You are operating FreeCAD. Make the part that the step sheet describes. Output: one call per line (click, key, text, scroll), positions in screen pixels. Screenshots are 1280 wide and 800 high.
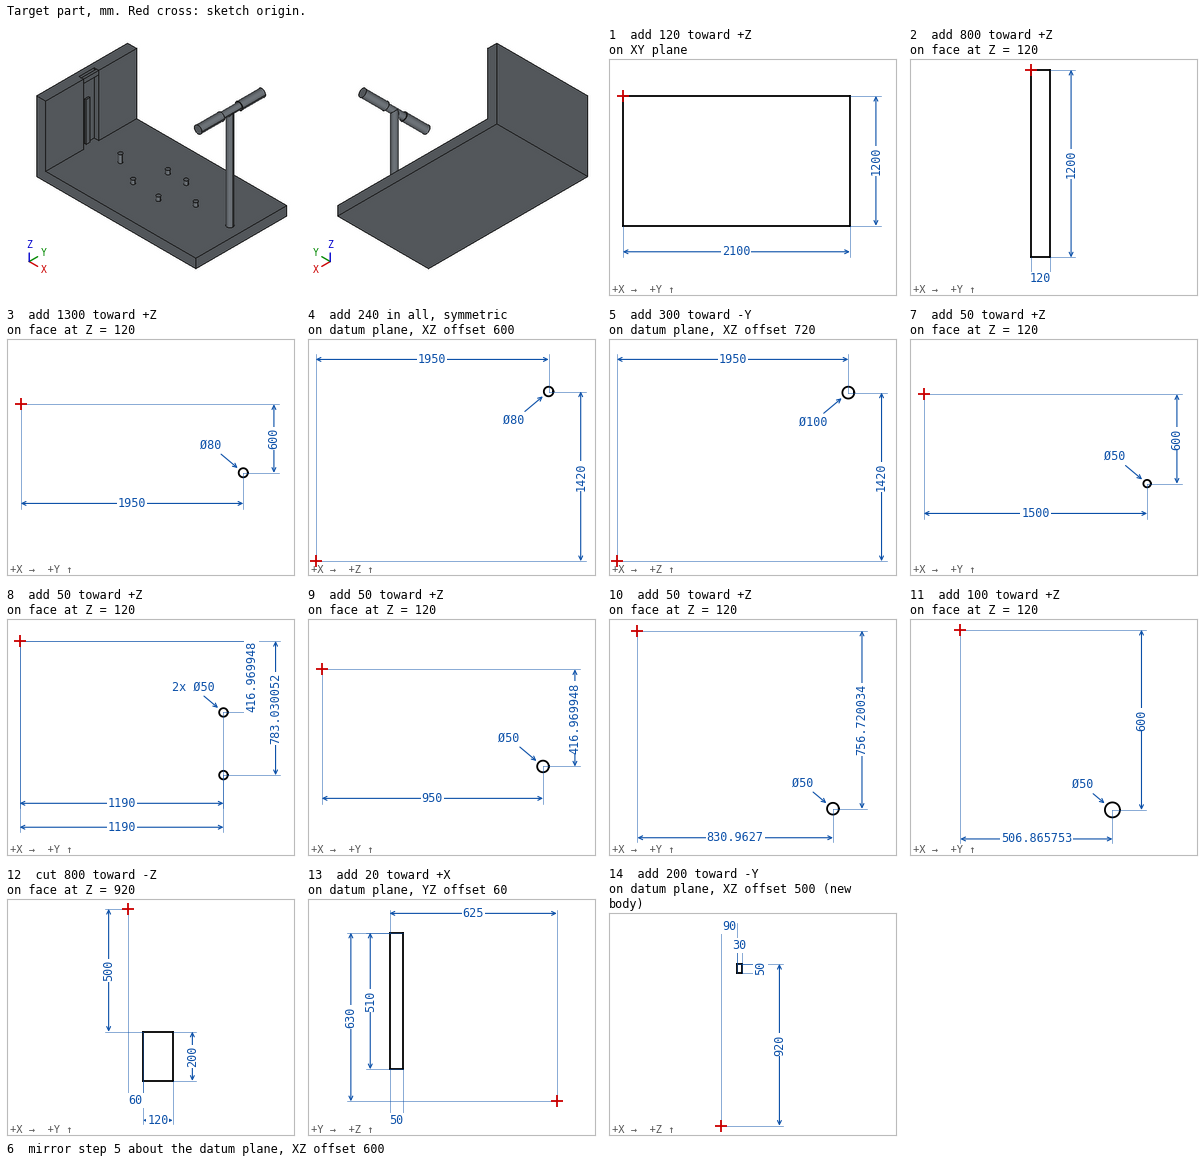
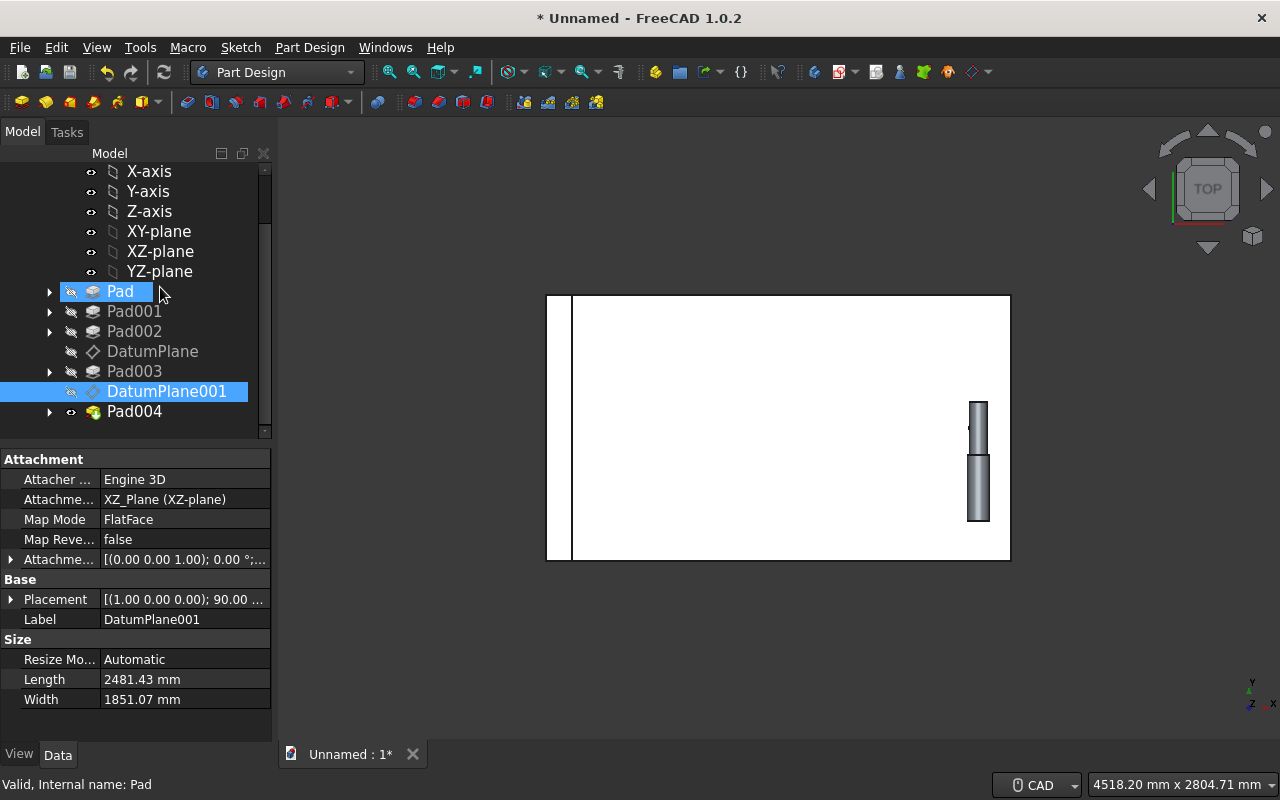
scroll(160, 287, up, 15)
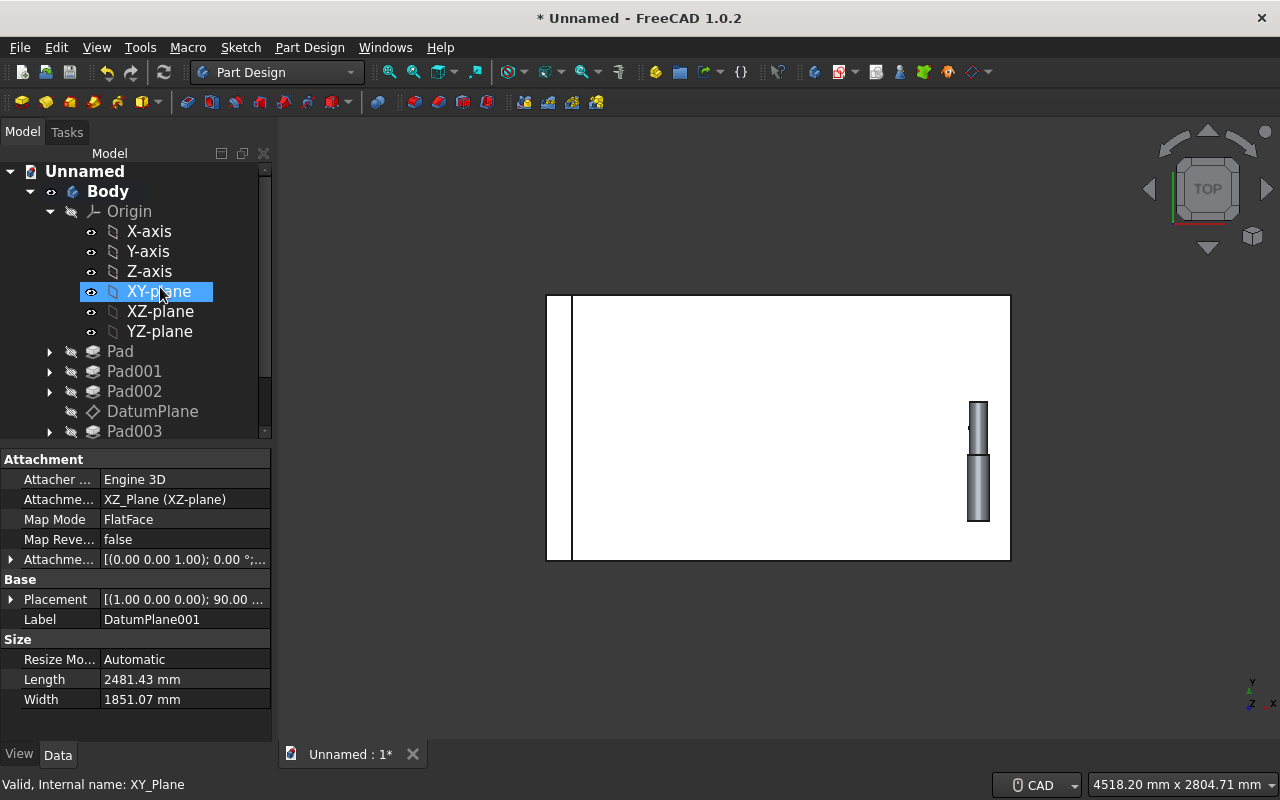
click(136, 312)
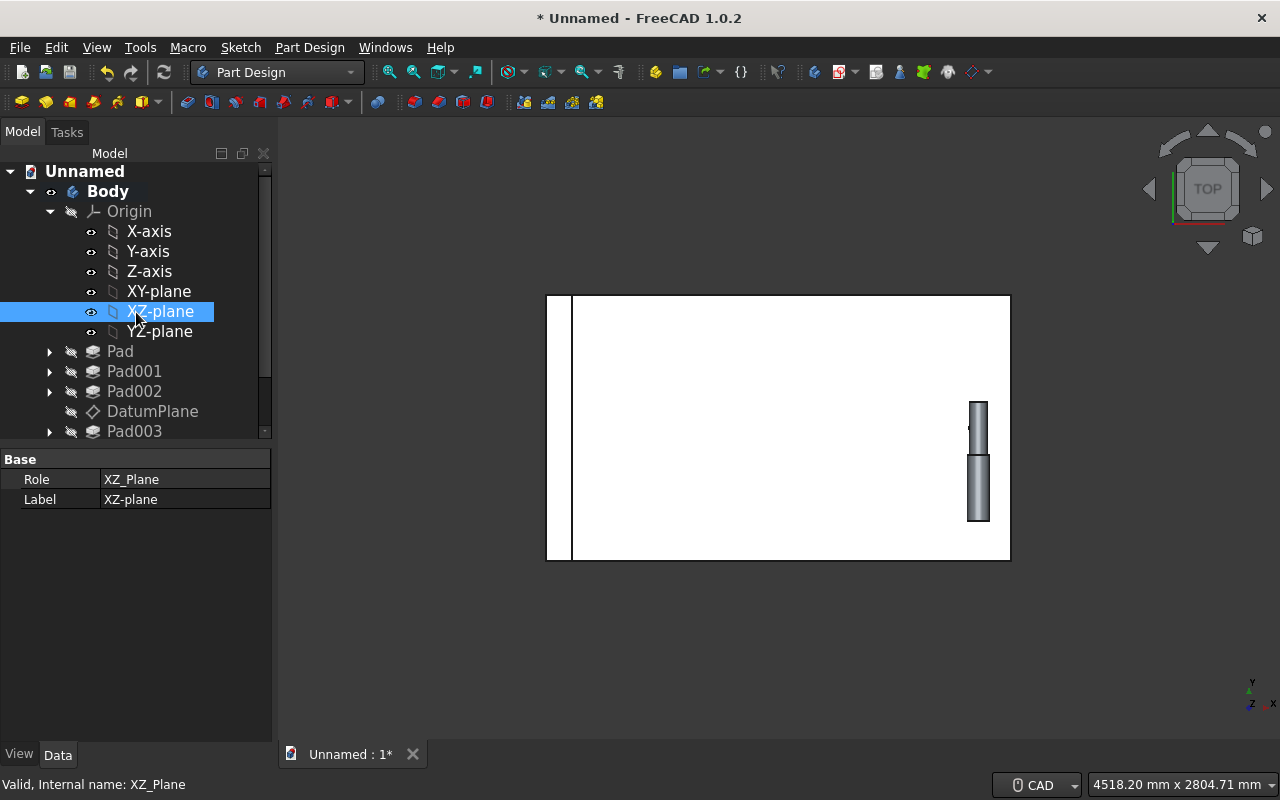
click(972, 72)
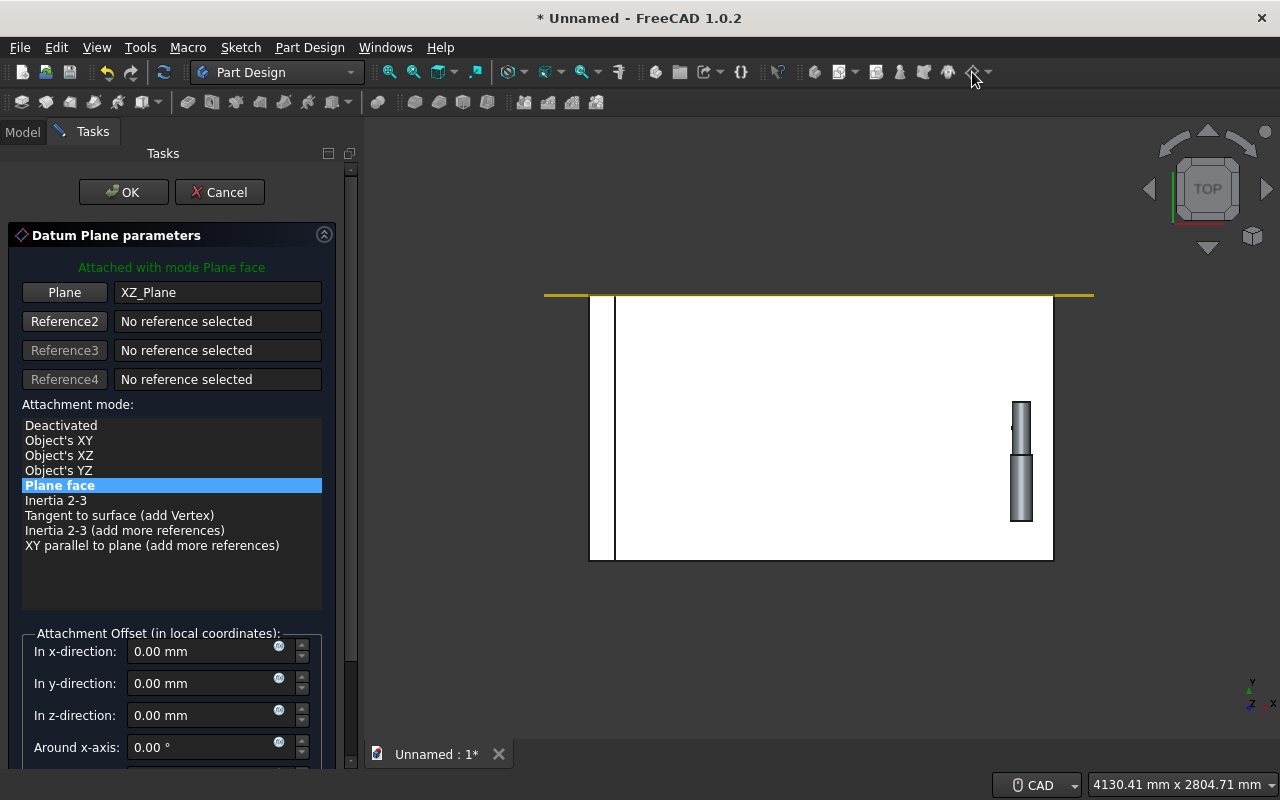
triple_click(210, 715)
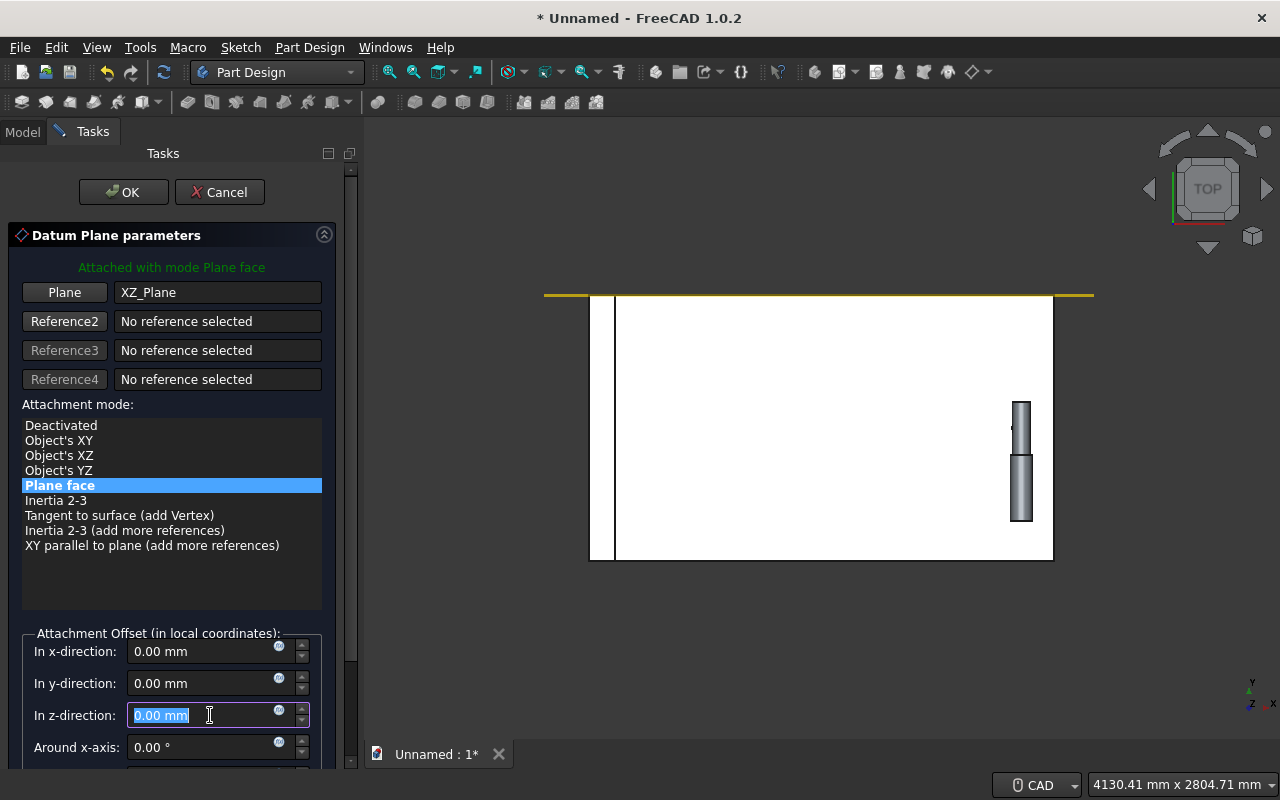
text(600)
key(Tab)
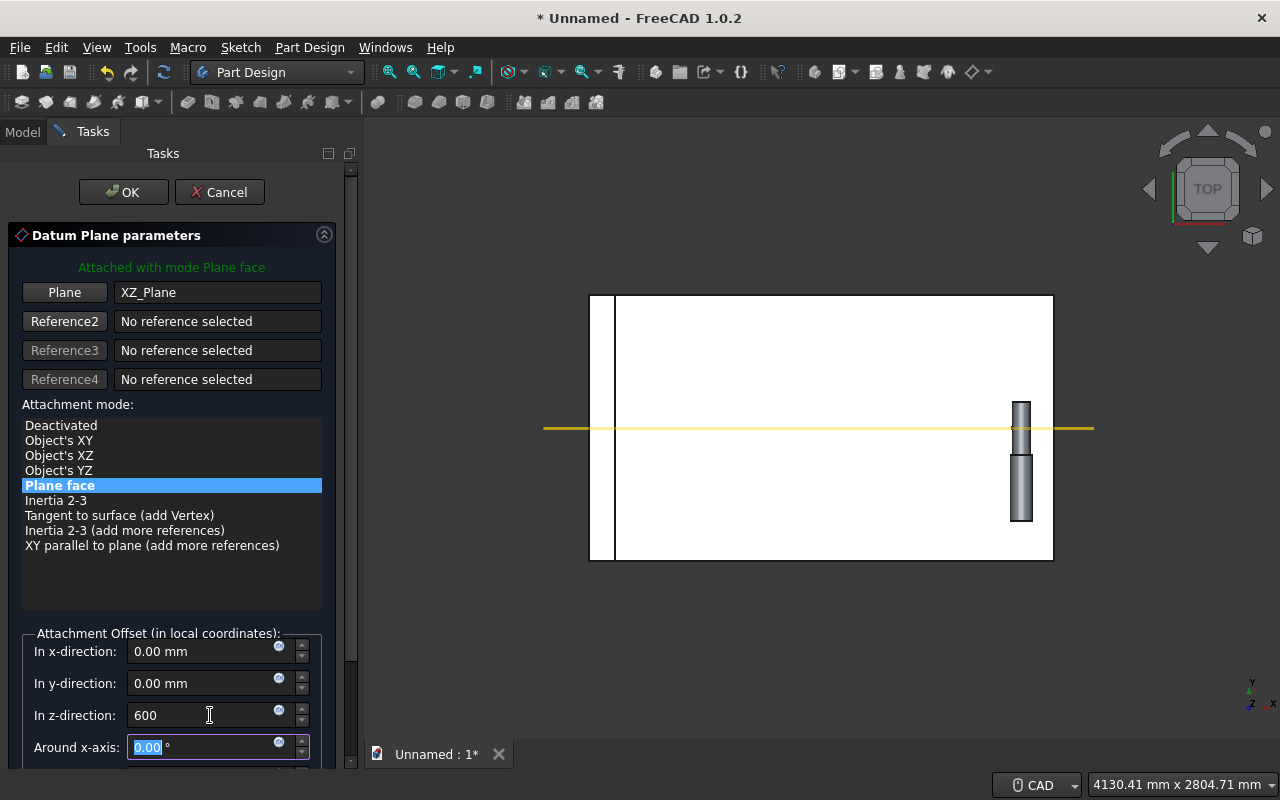
click(124, 192)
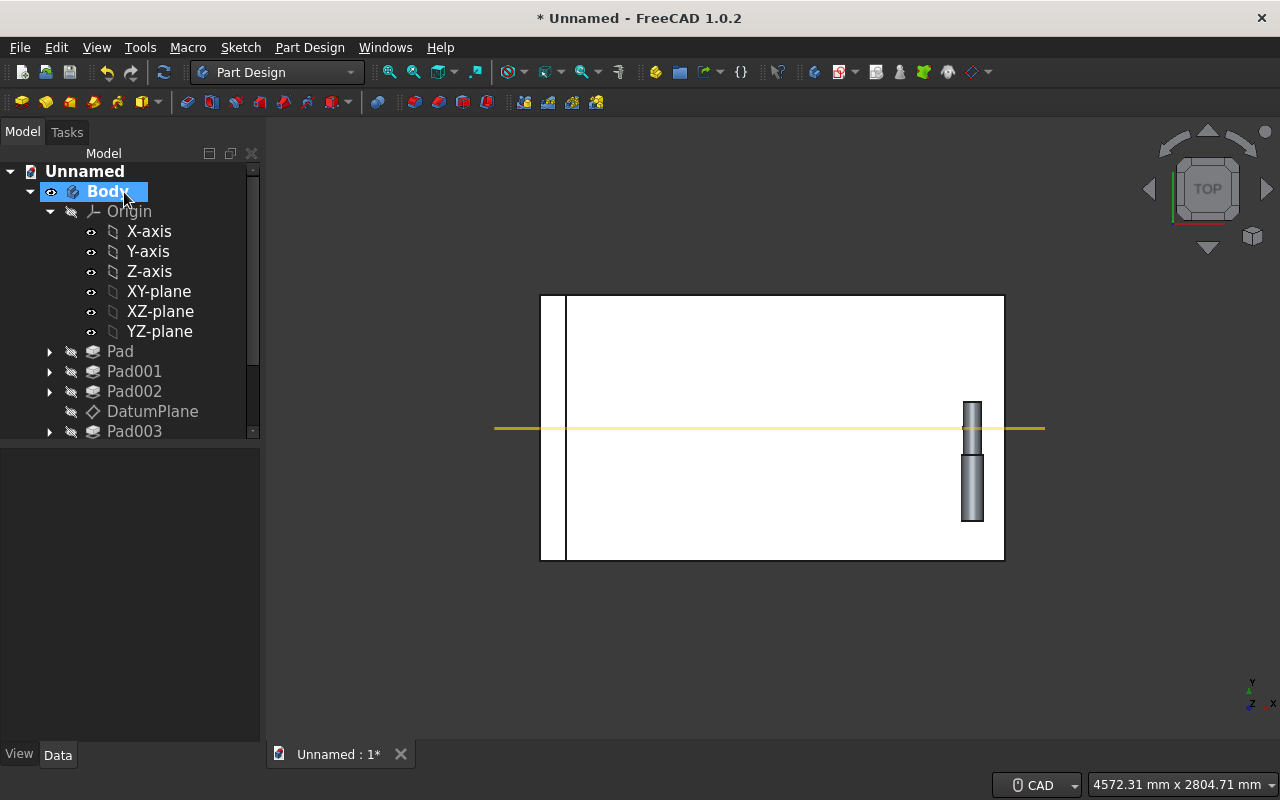
scroll(100, 307, down, 3)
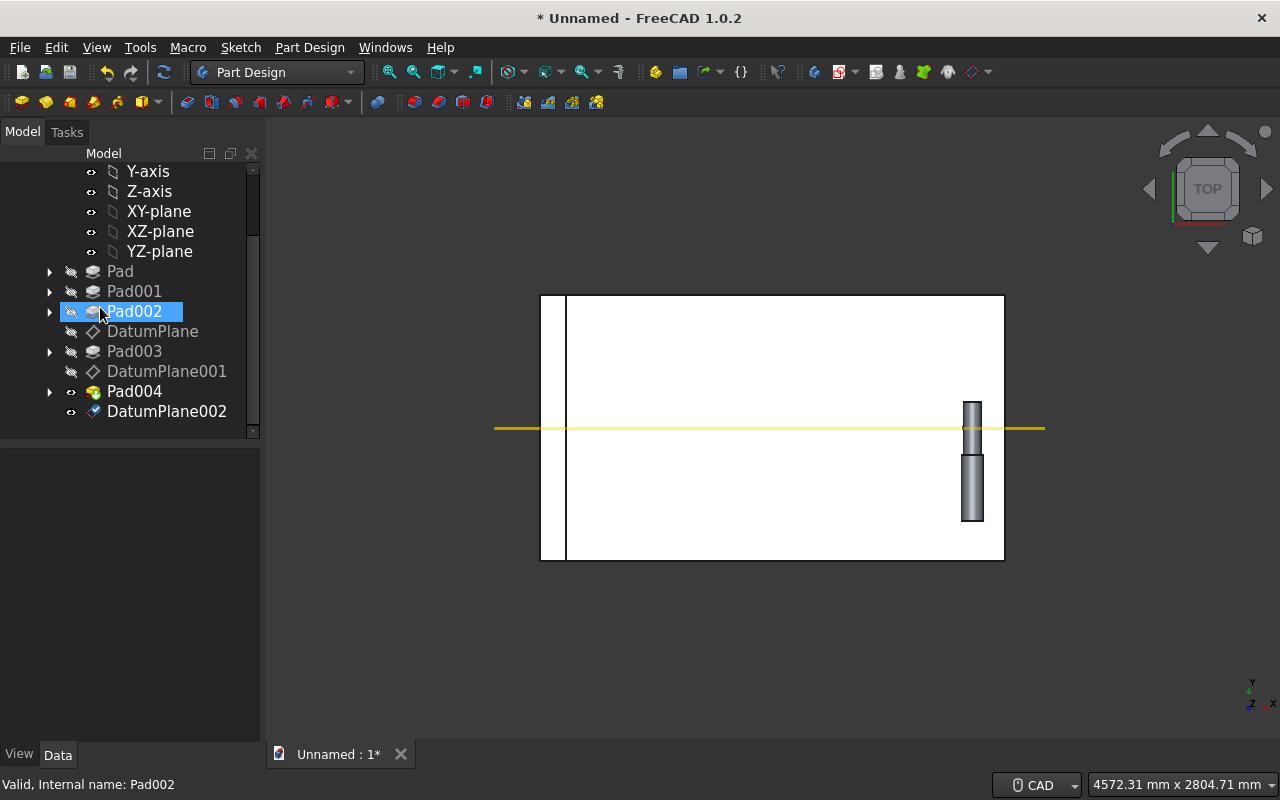
click(116, 392)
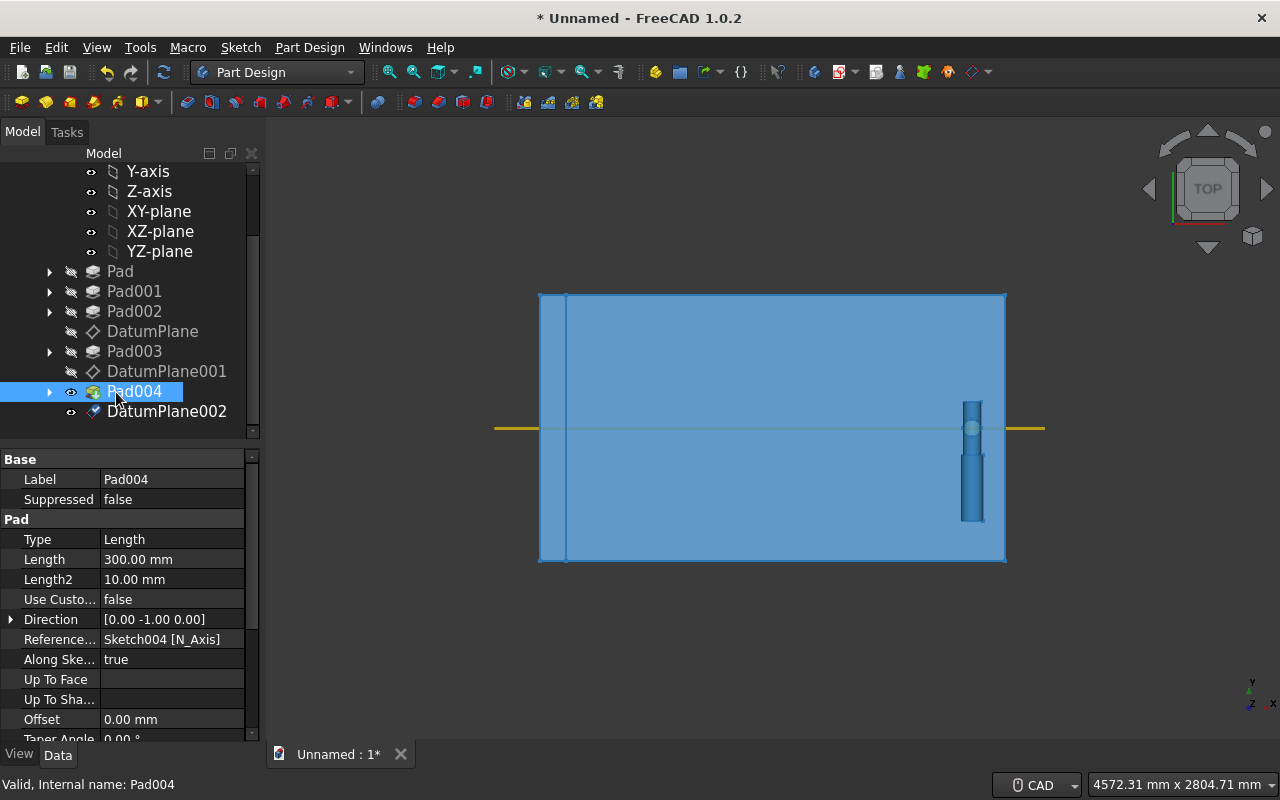
click(524, 102)